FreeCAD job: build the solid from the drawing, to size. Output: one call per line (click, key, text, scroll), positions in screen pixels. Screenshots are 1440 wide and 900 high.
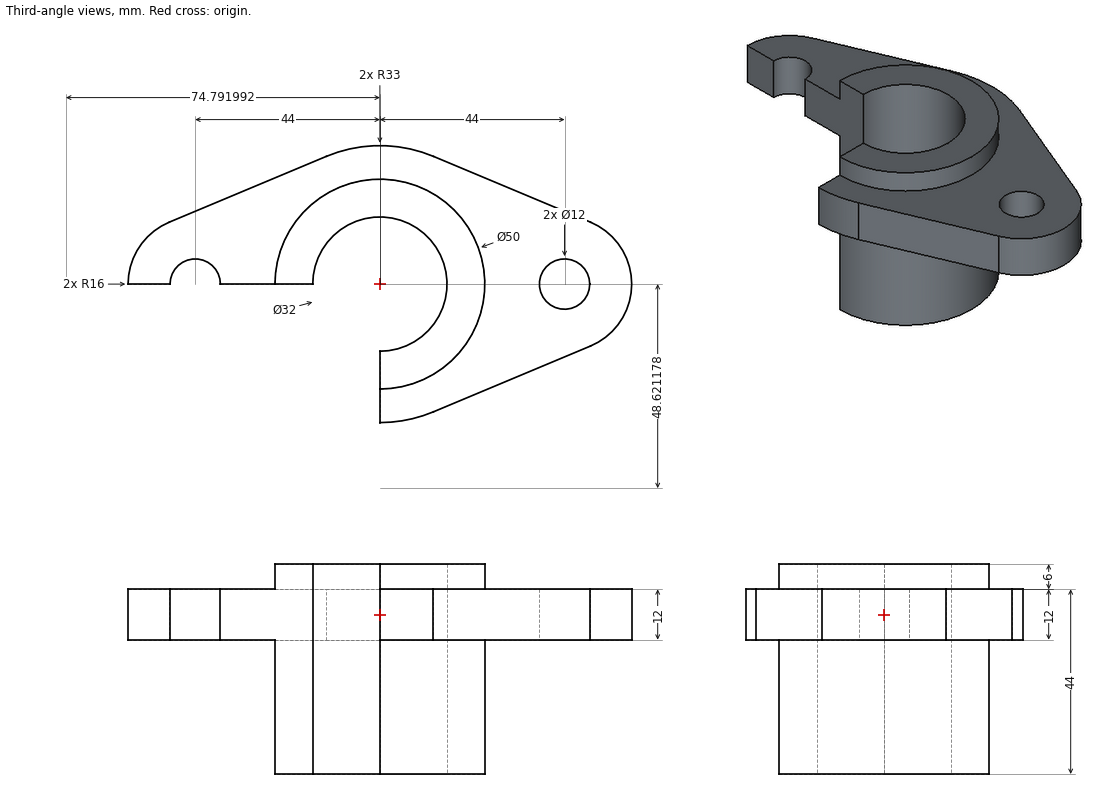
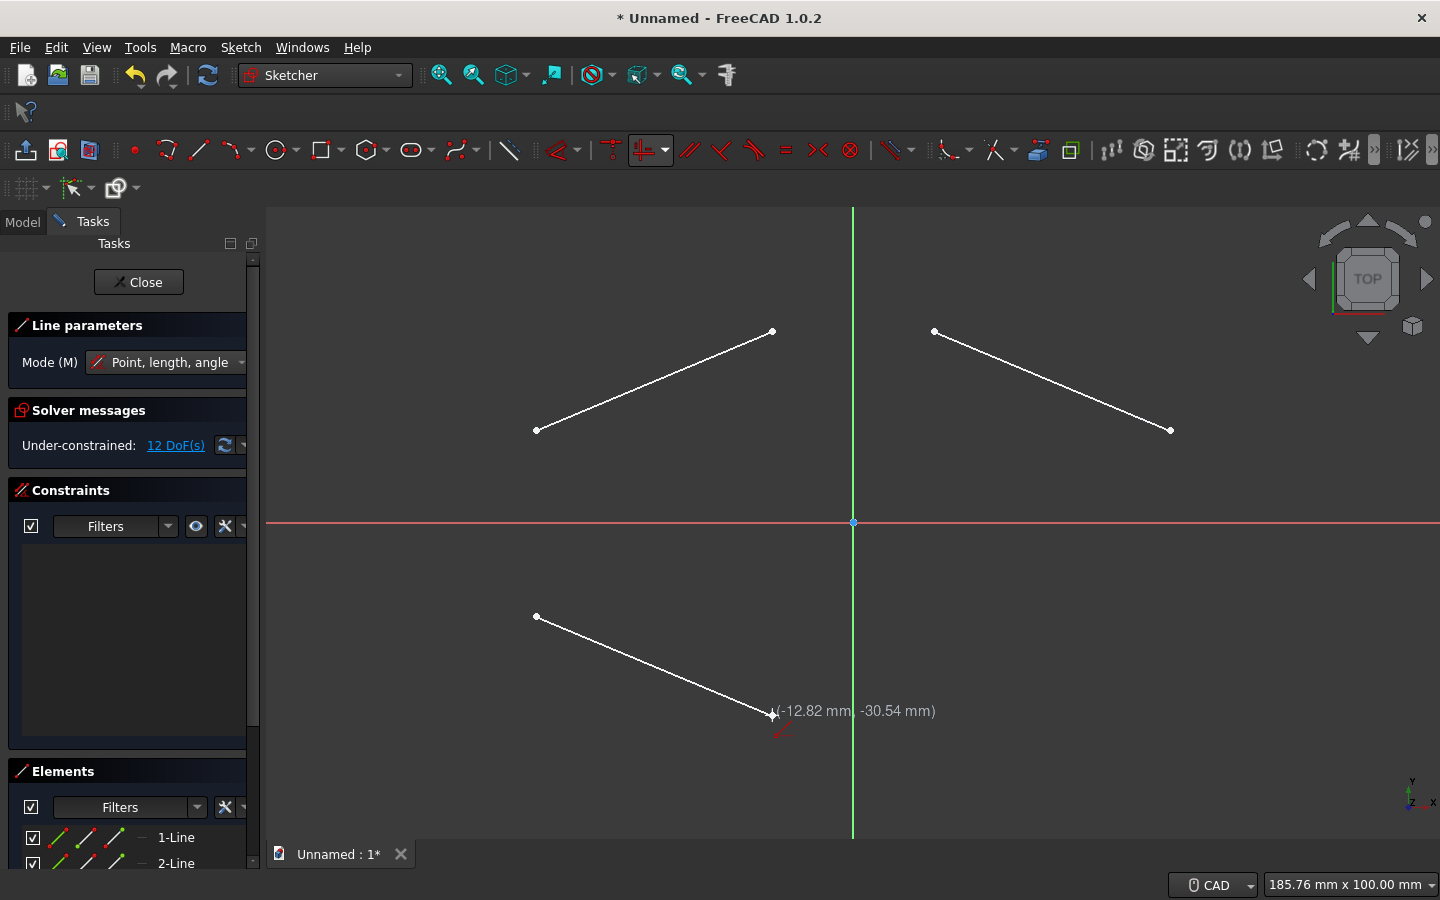
click(934, 715)
click(1170, 616)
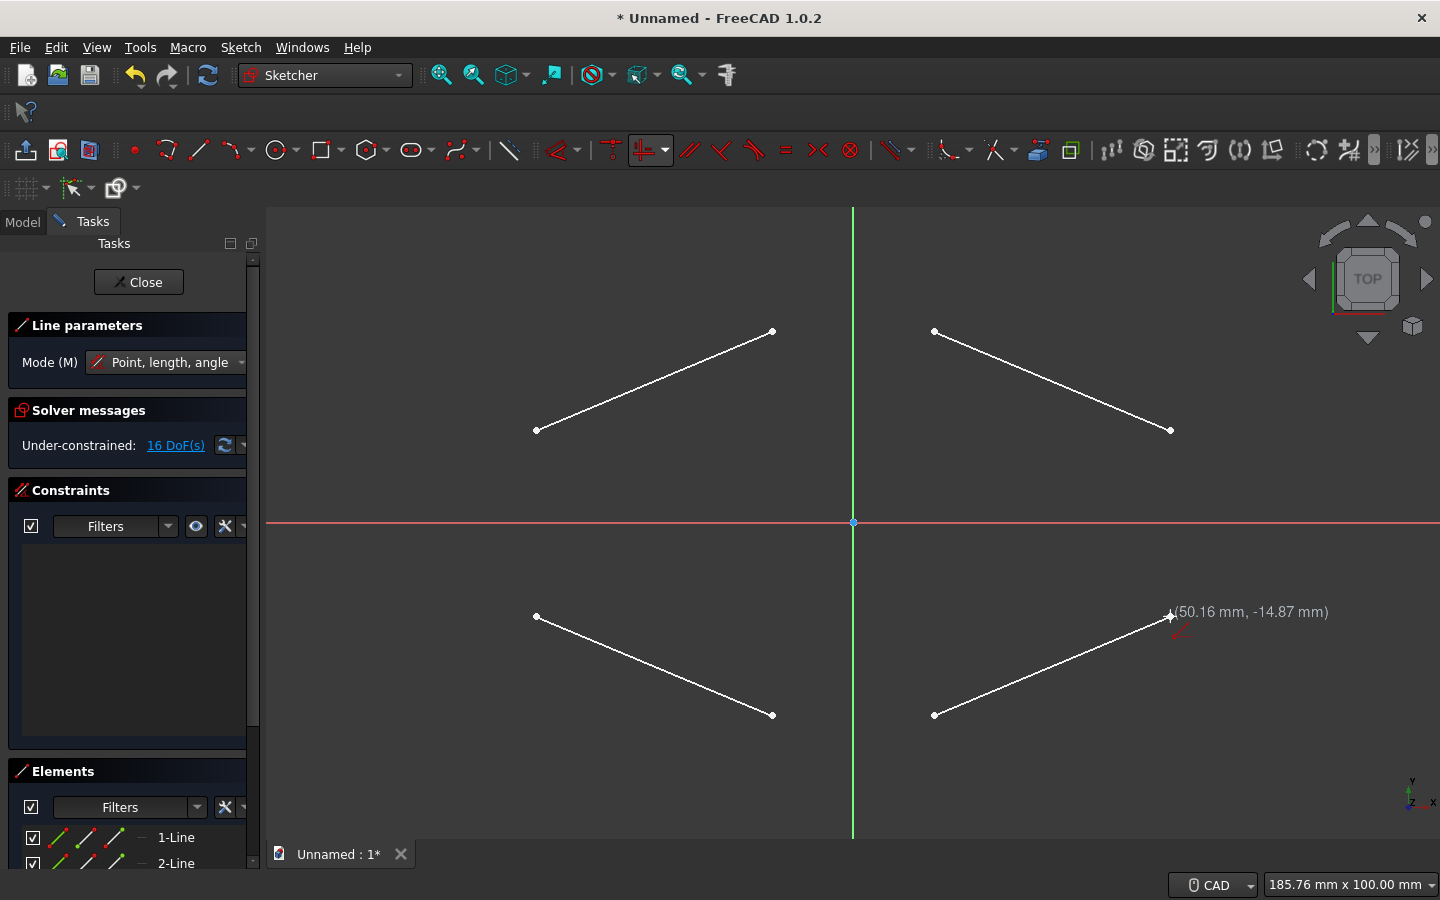
click(232, 150)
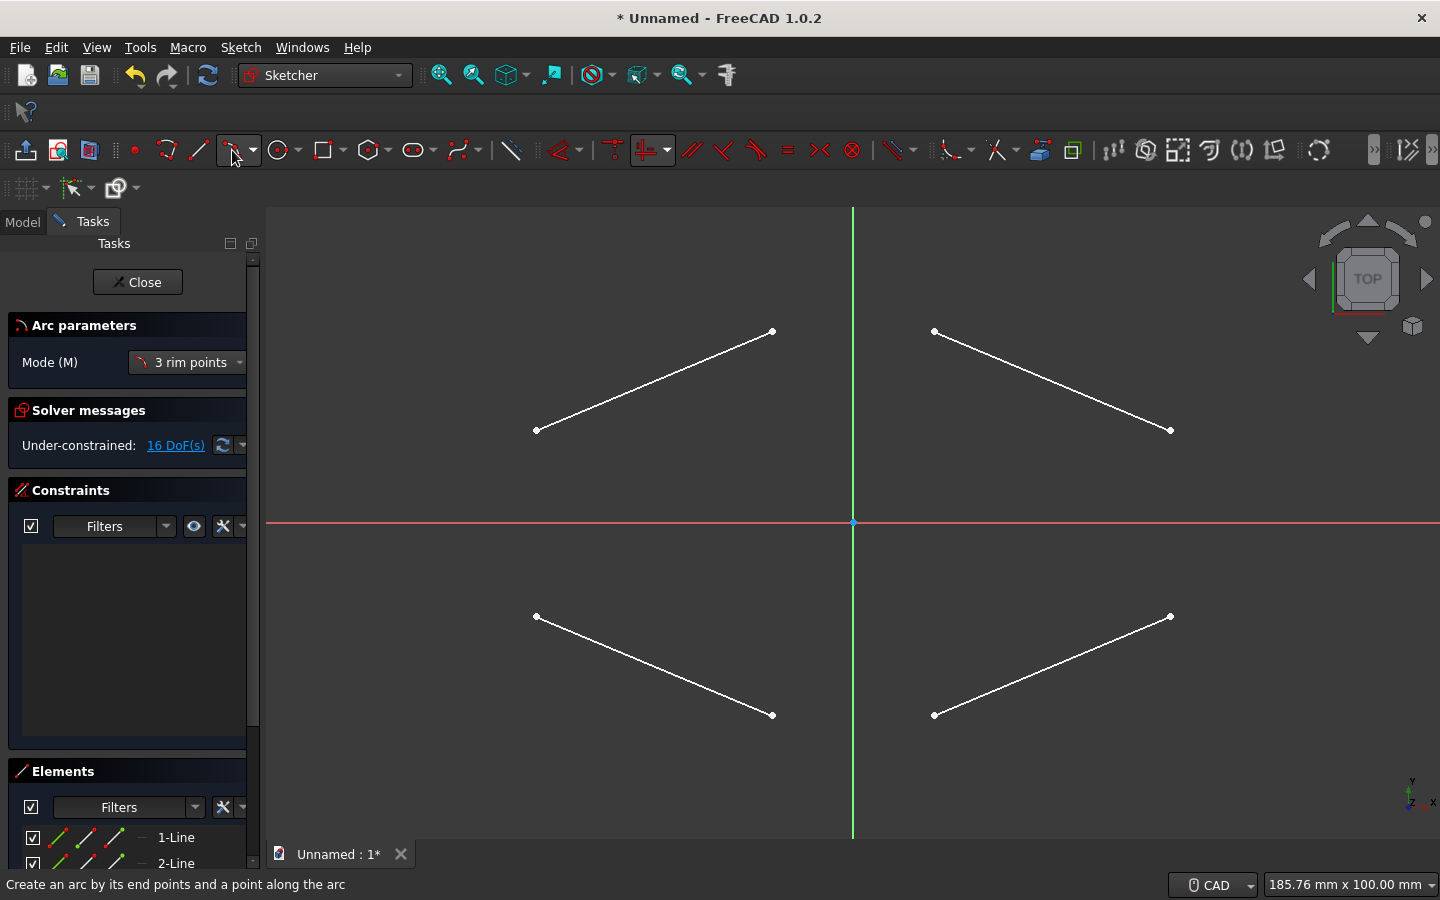
click(934, 332)
click(772, 332)
click(870, 315)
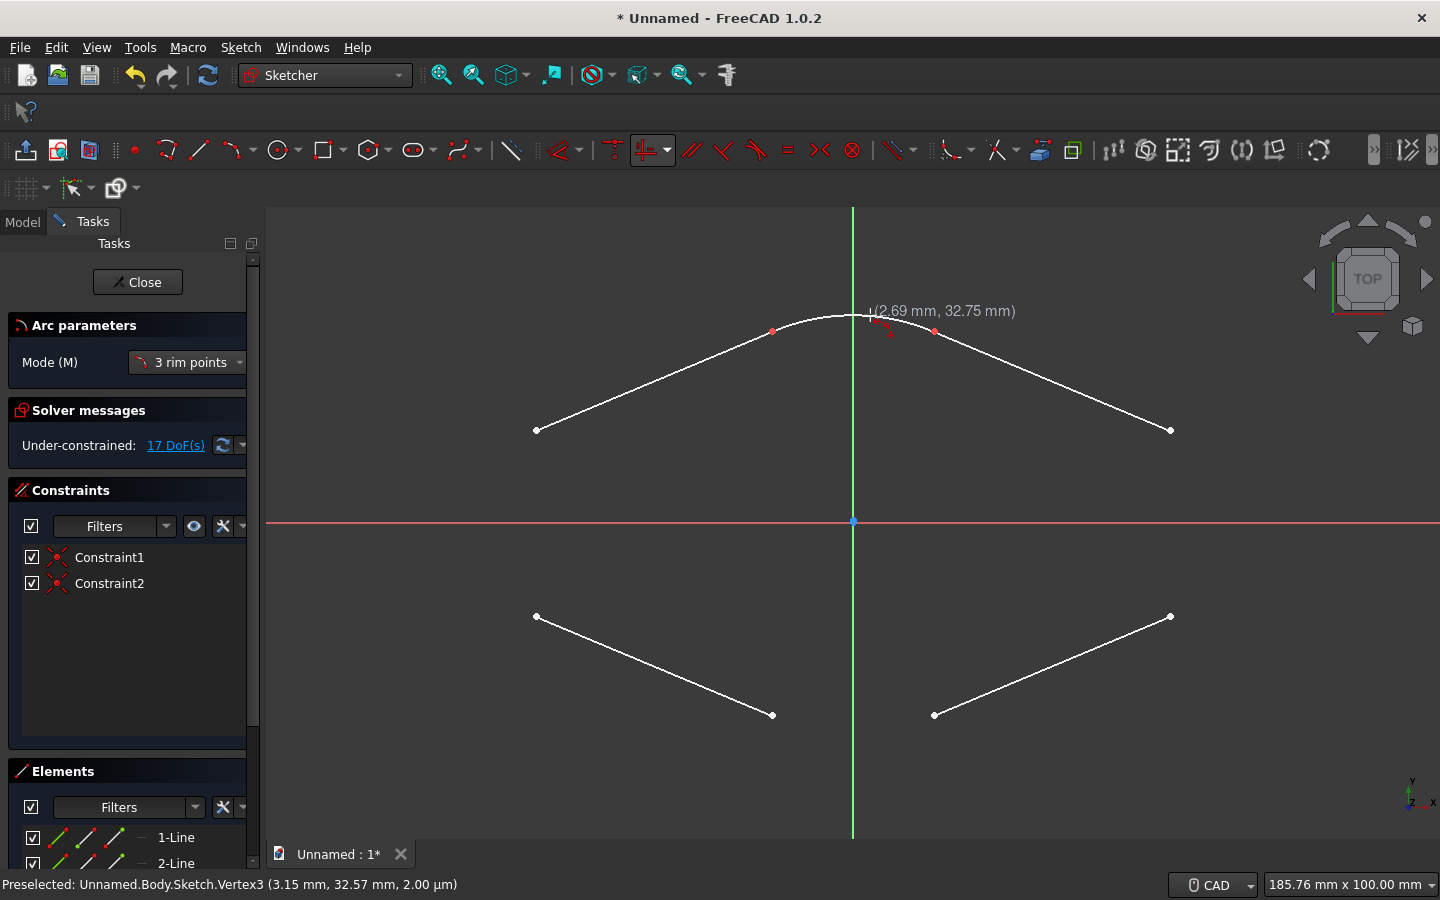
click(536, 431)
click(536, 617)
click(477, 499)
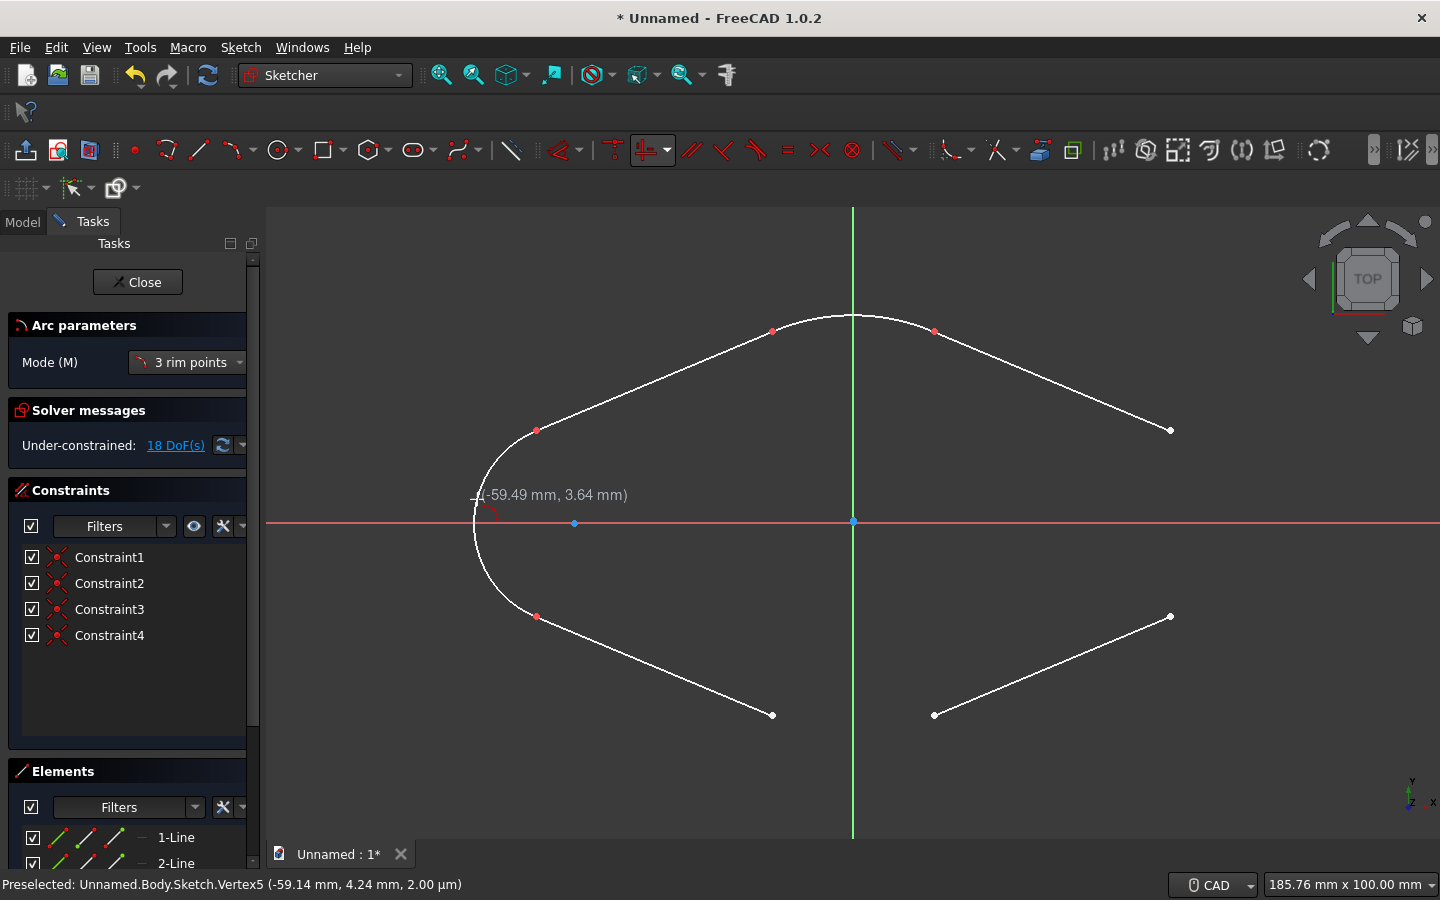
click(772, 716)
click(934, 716)
click(836, 731)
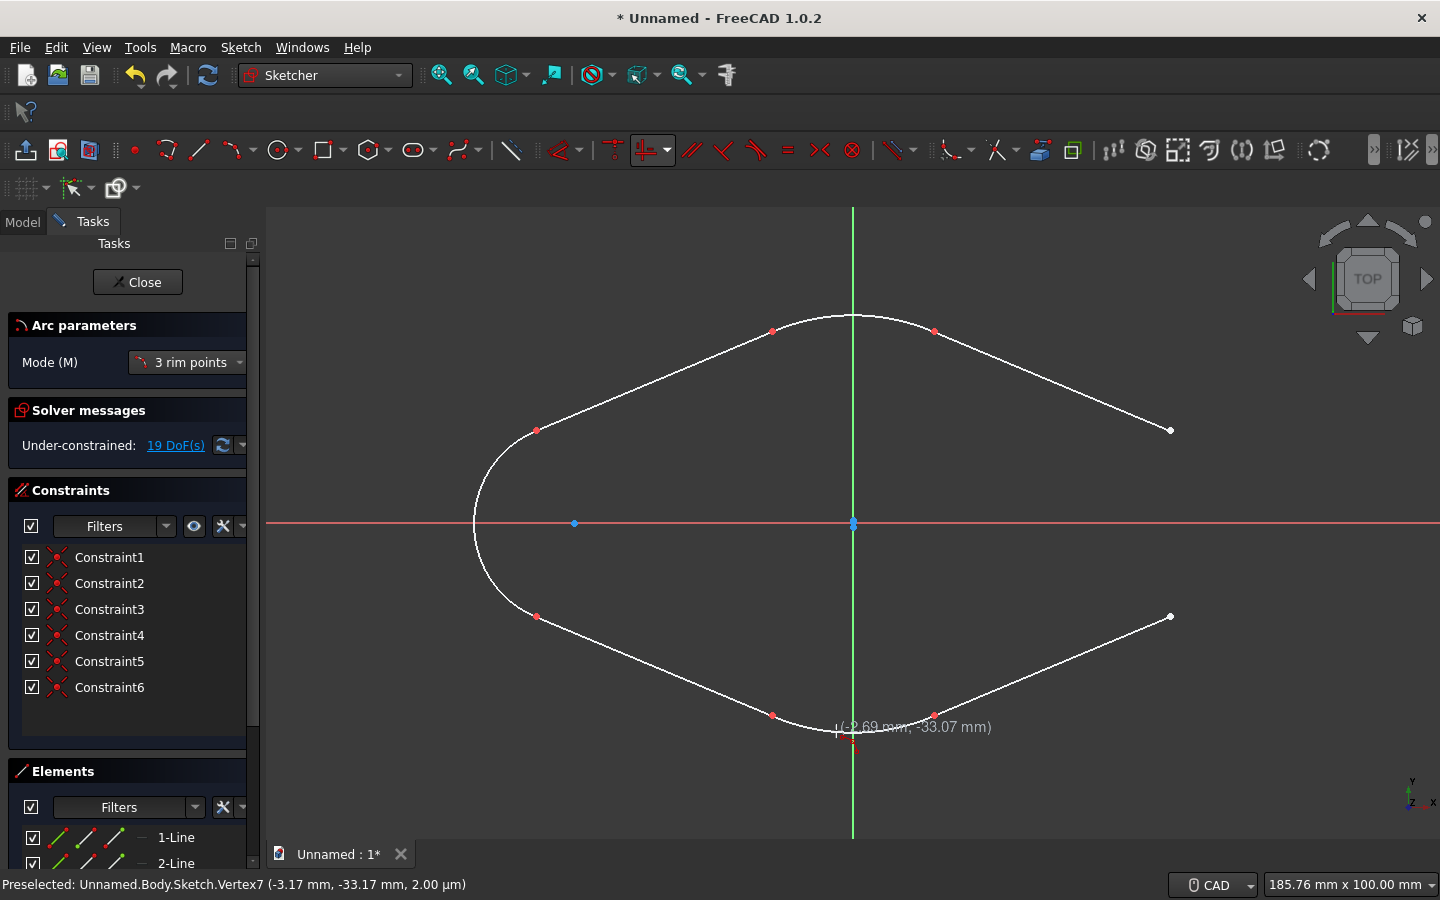
click(1170, 617)
click(1170, 431)
click(1229, 547)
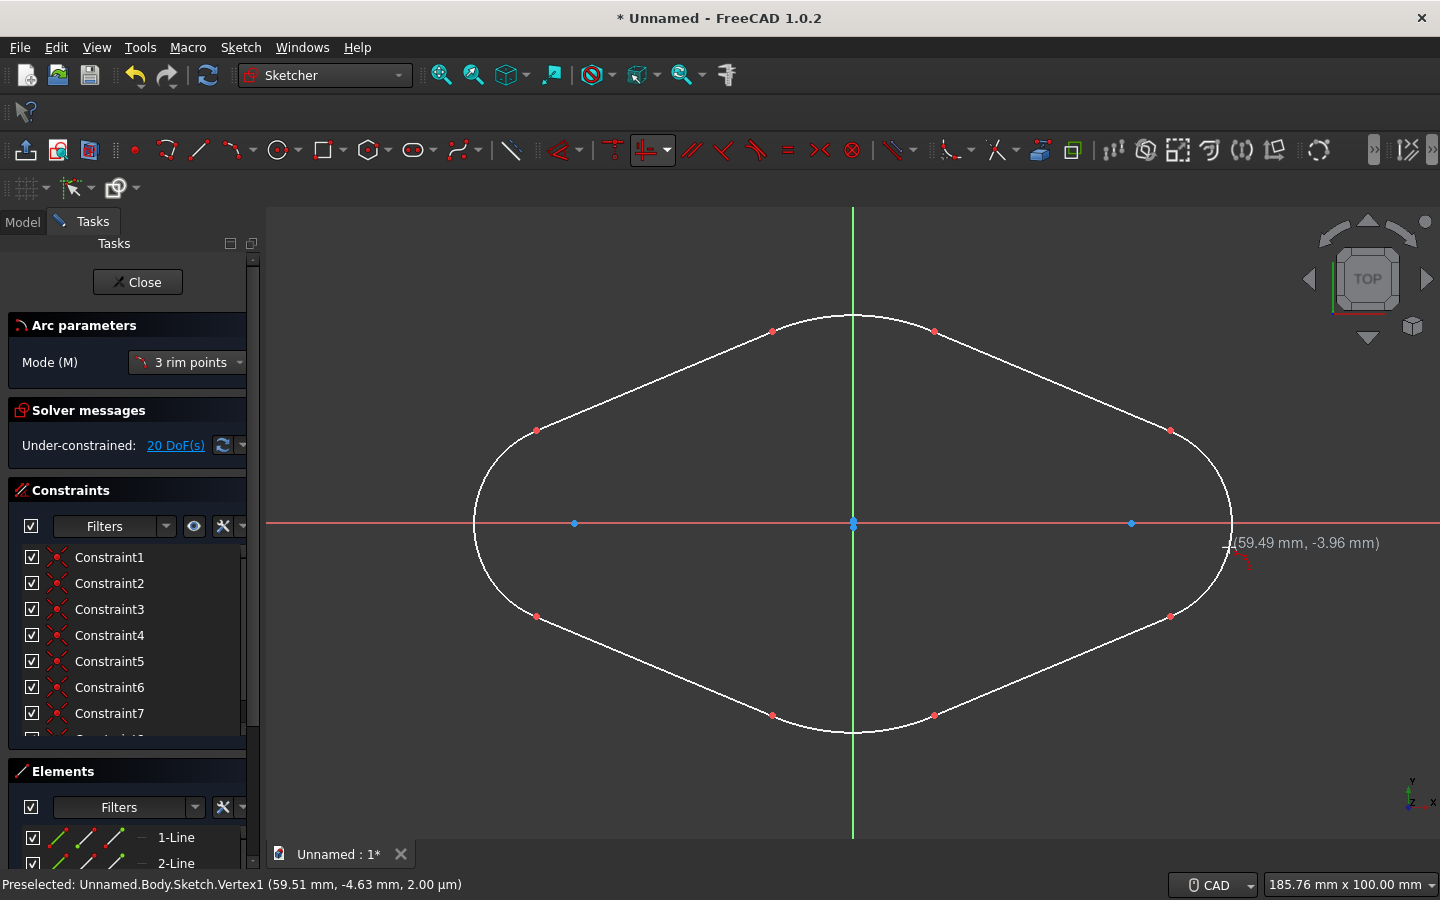
click(278, 150)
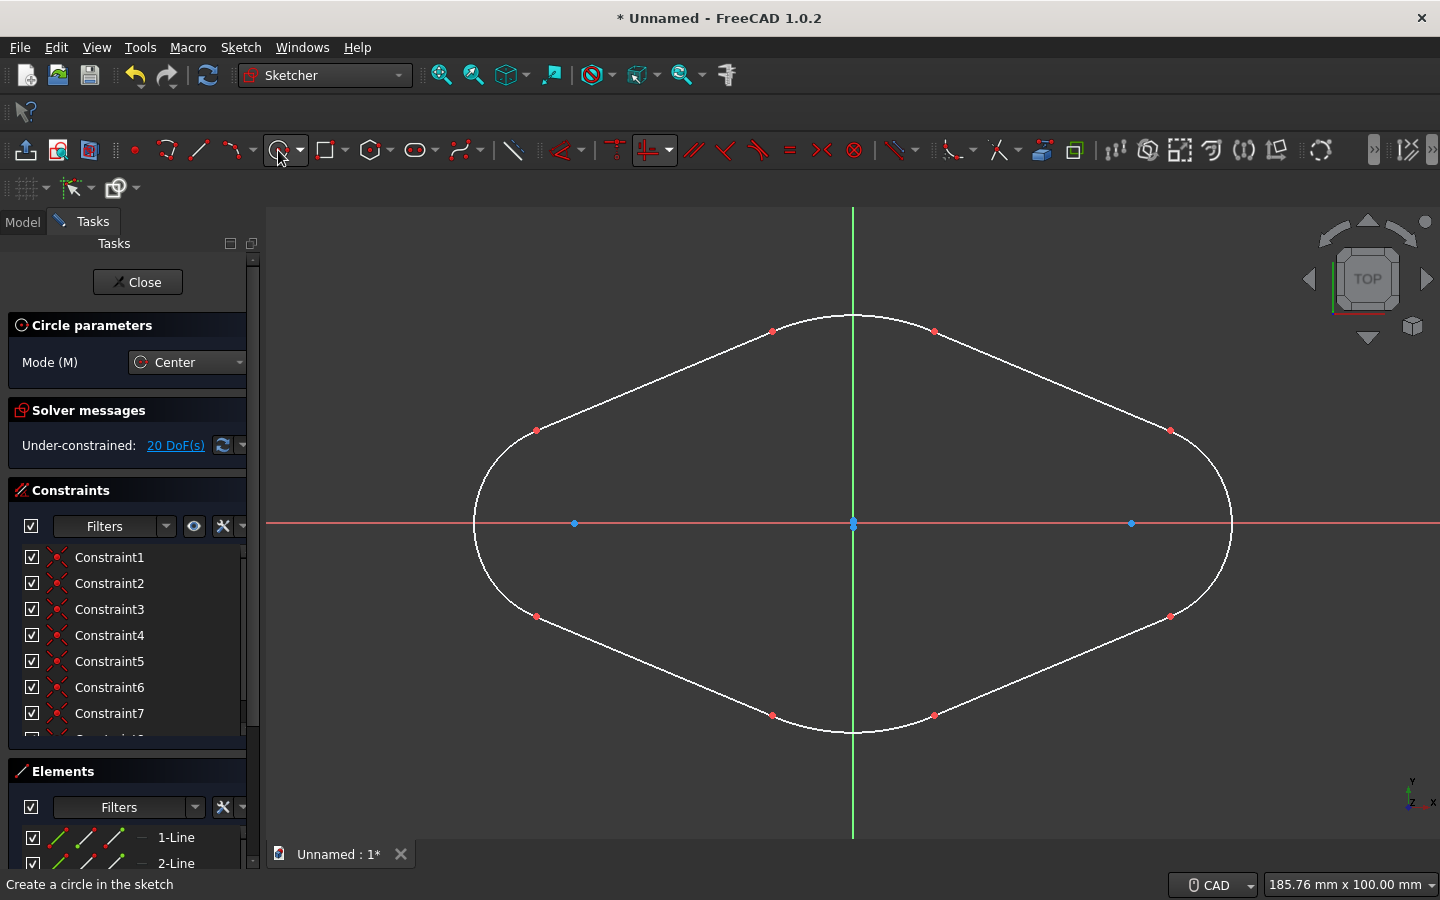
click(1131, 523)
move(1158, 496)